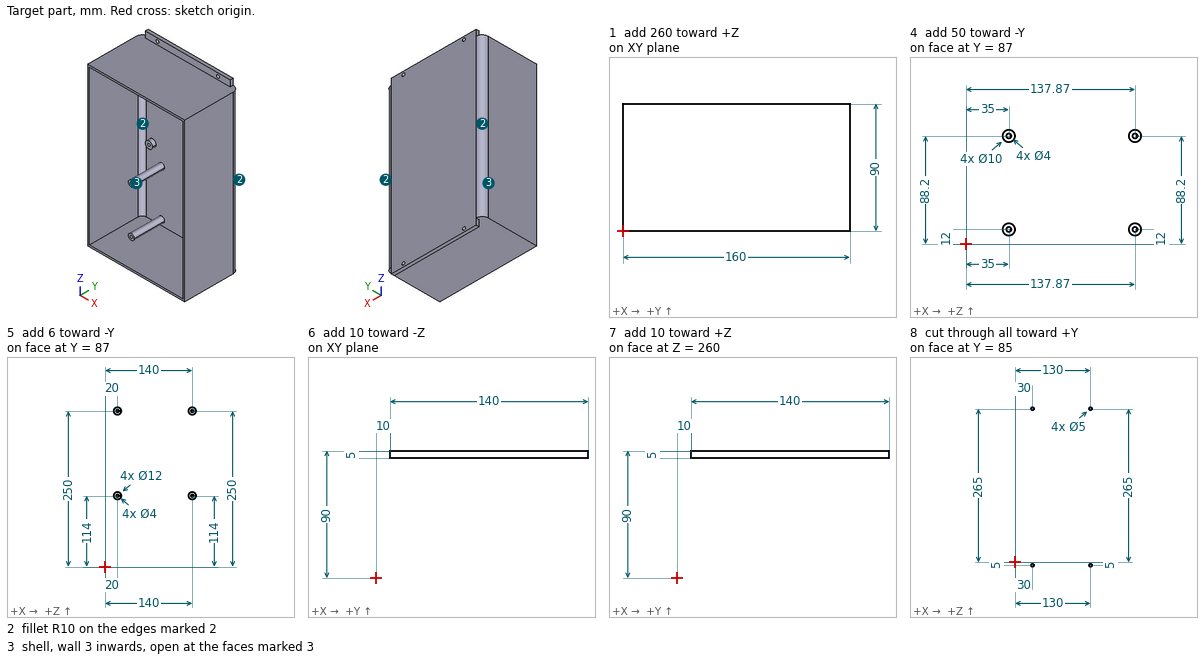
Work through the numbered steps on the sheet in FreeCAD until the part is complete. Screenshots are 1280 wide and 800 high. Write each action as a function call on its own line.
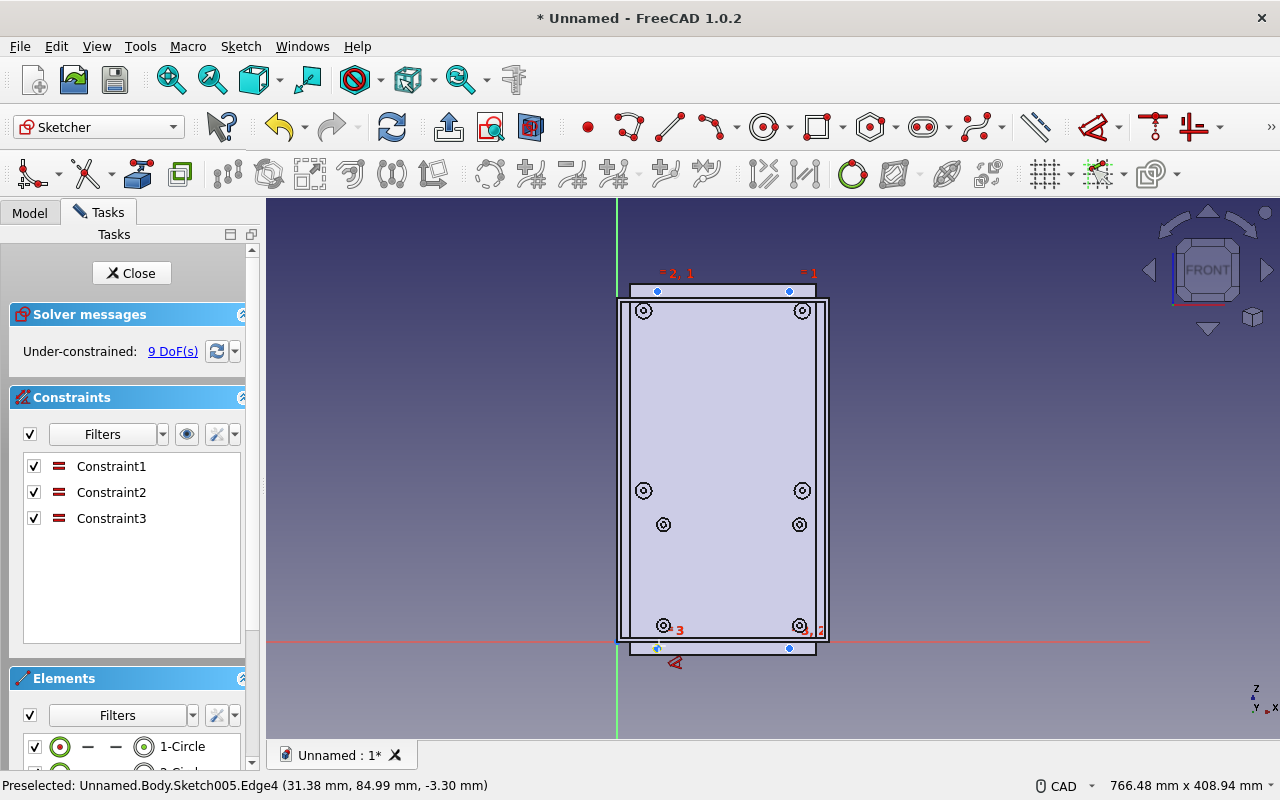
scroll(792, 289, up, 9)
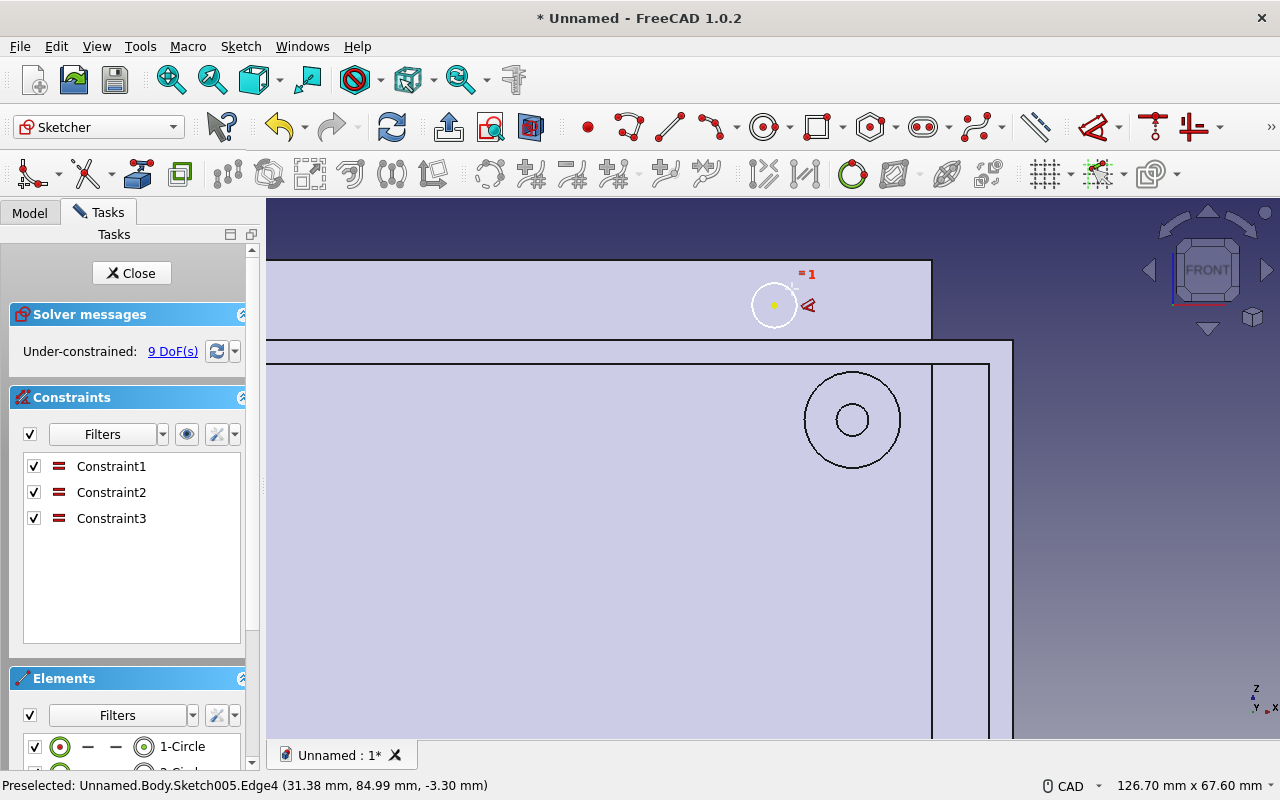
click(790, 290)
click(813, 267)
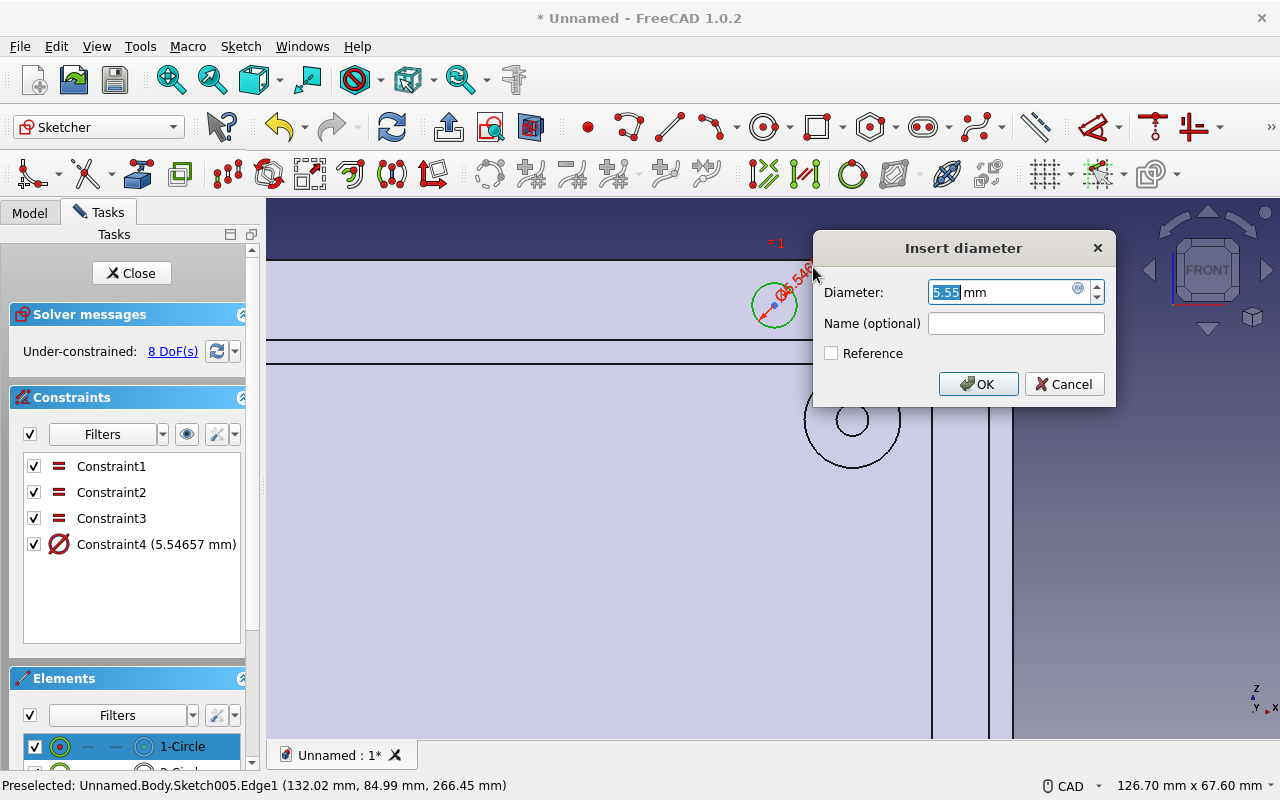
text(5)
key(Return)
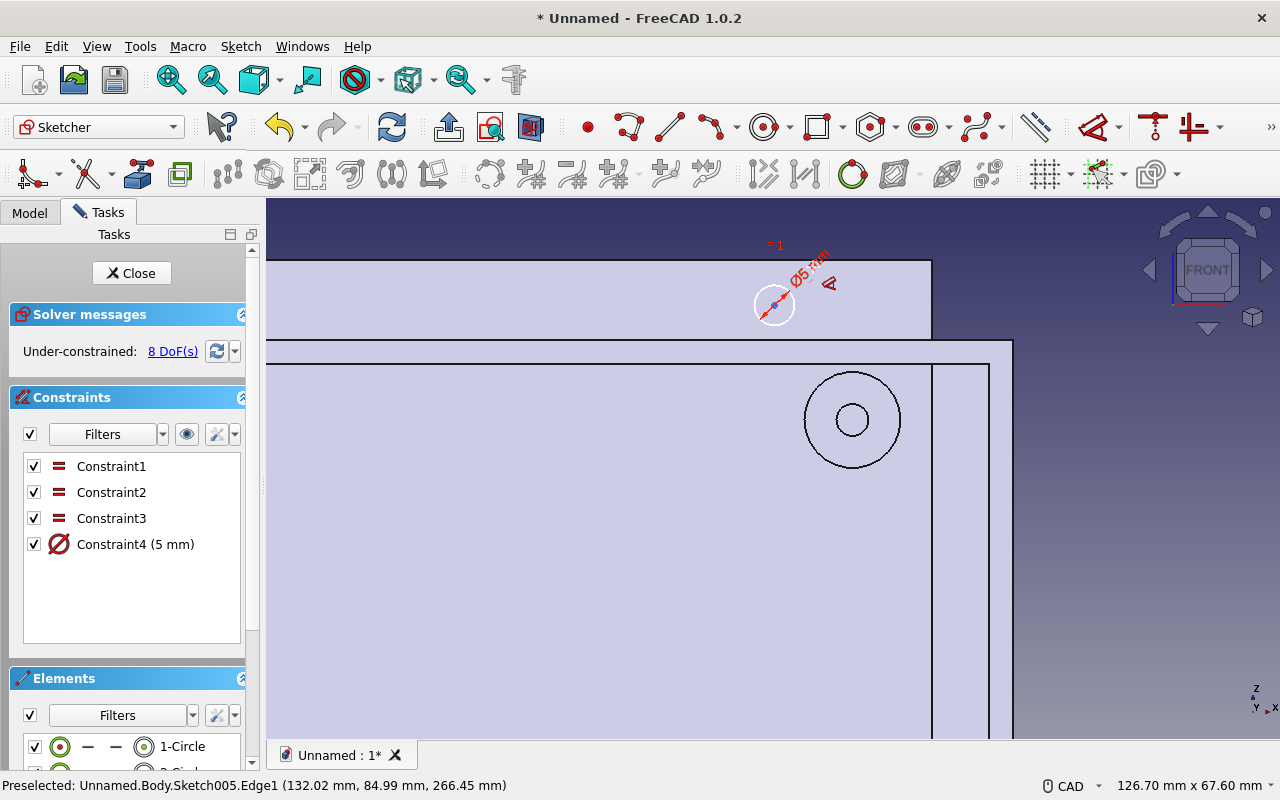
scroll(792, 288, down, 9)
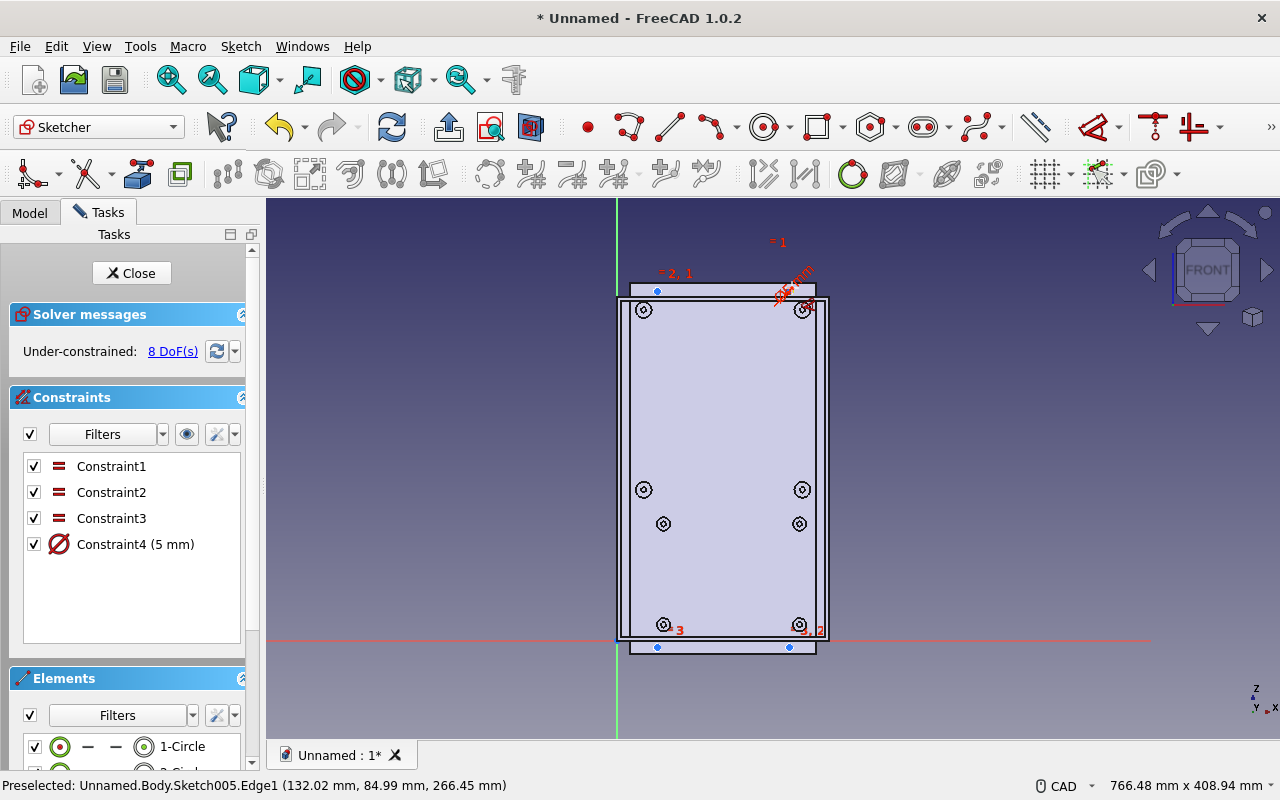
scroll(789, 648, up, 9)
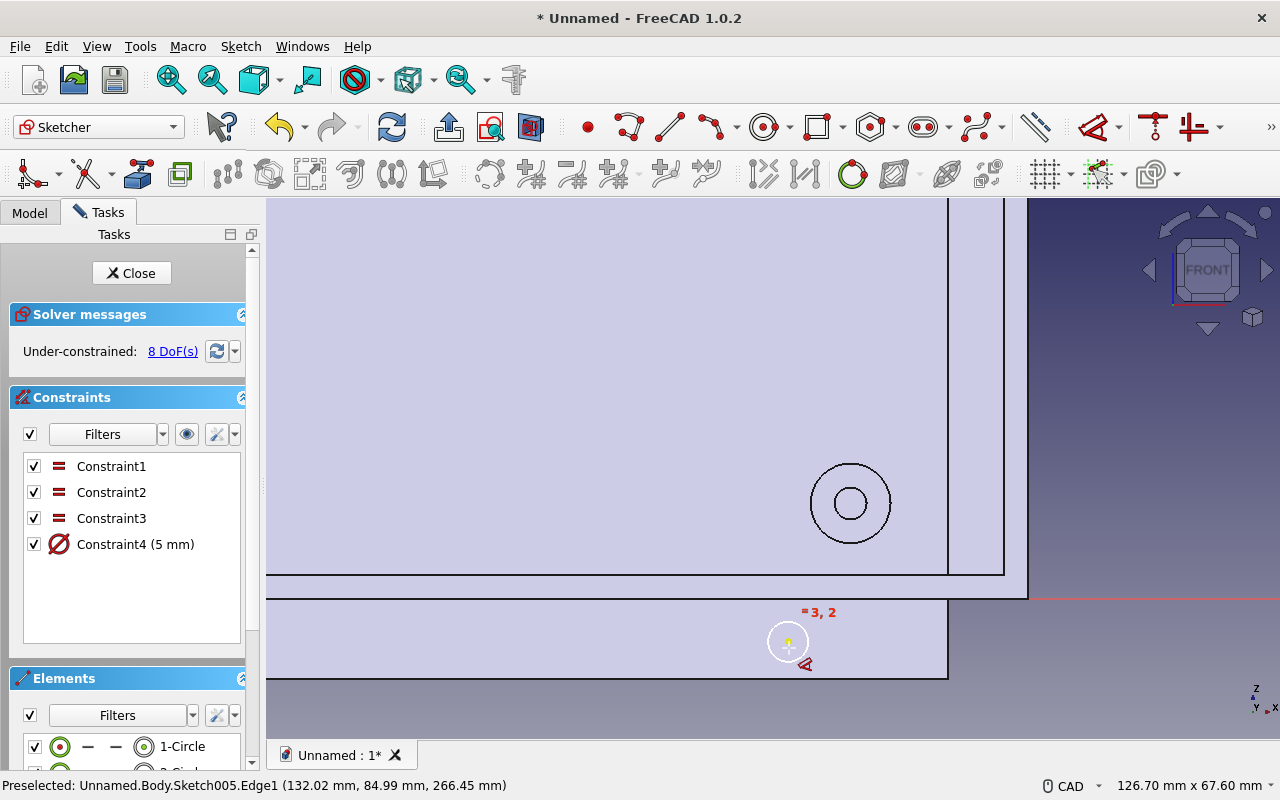
click(788, 642)
click(822, 621)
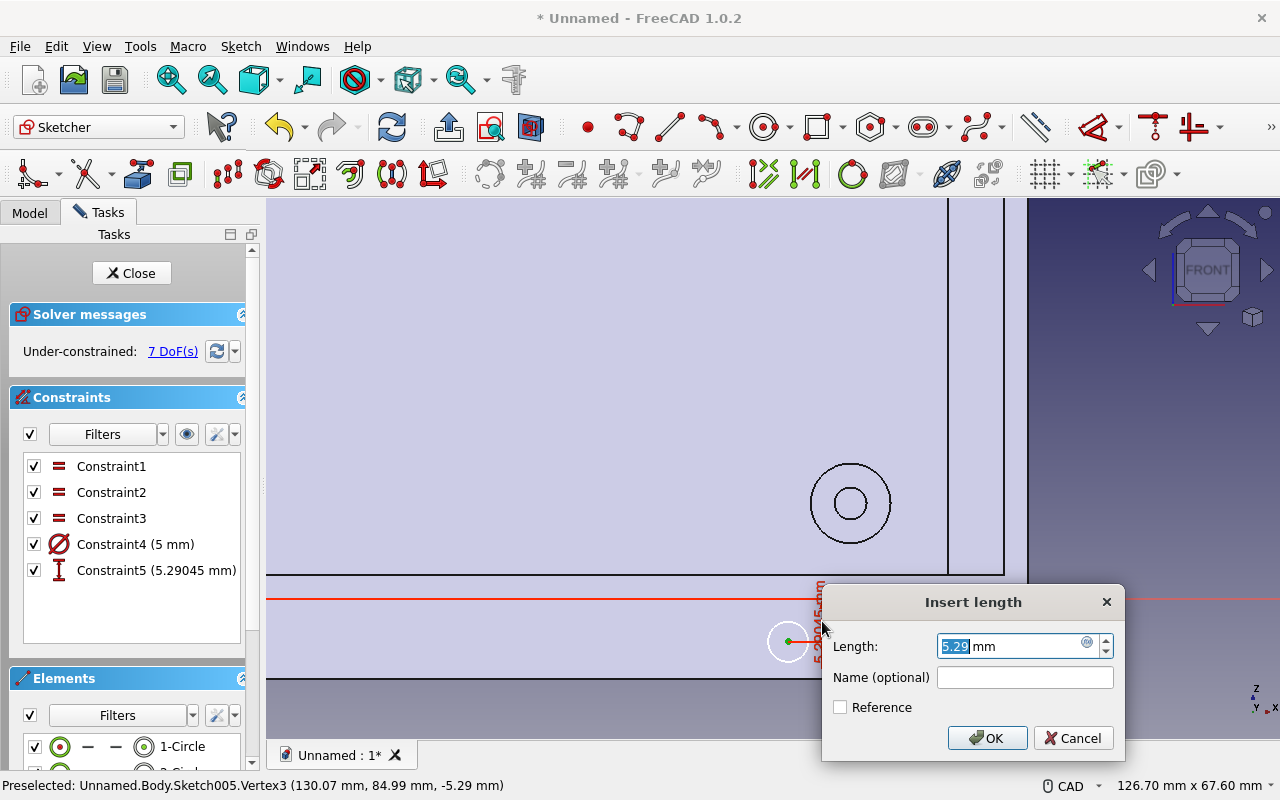
text(5)
key(Return)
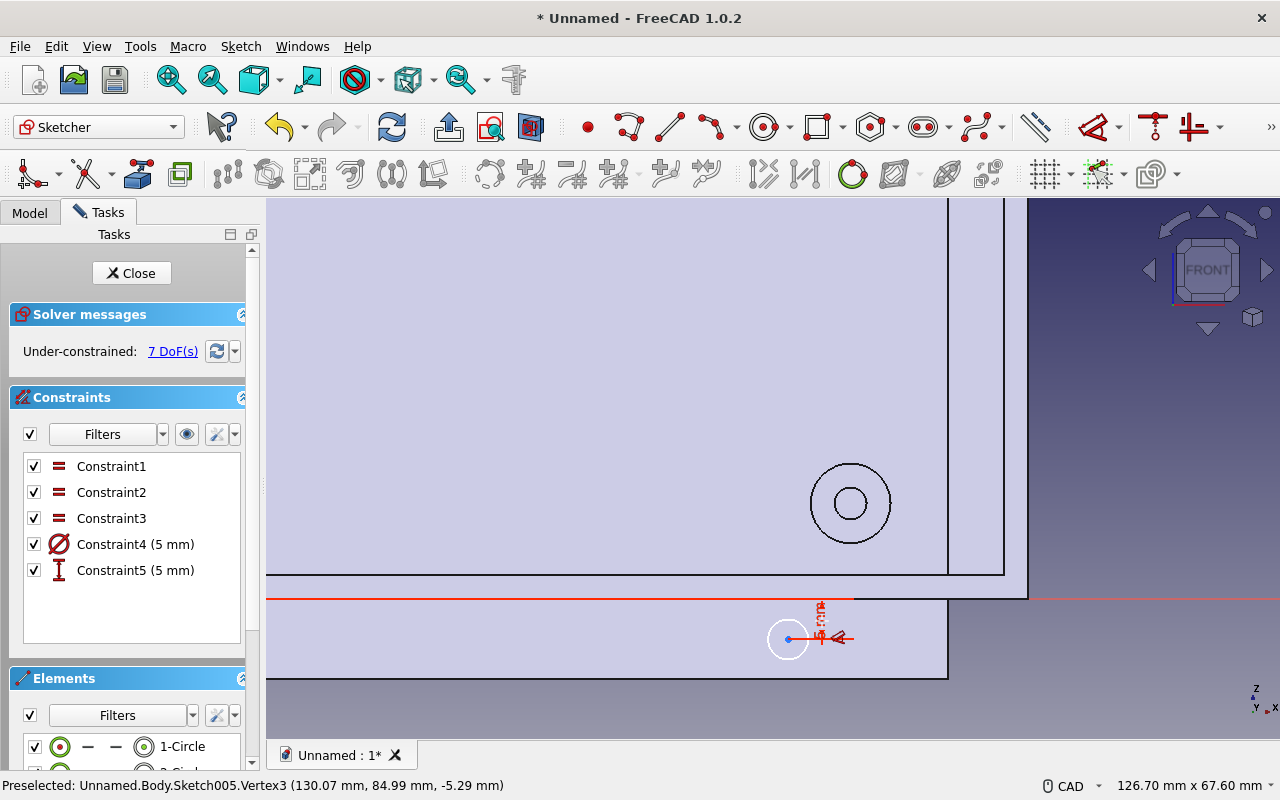
scroll(789, 649, down, 9)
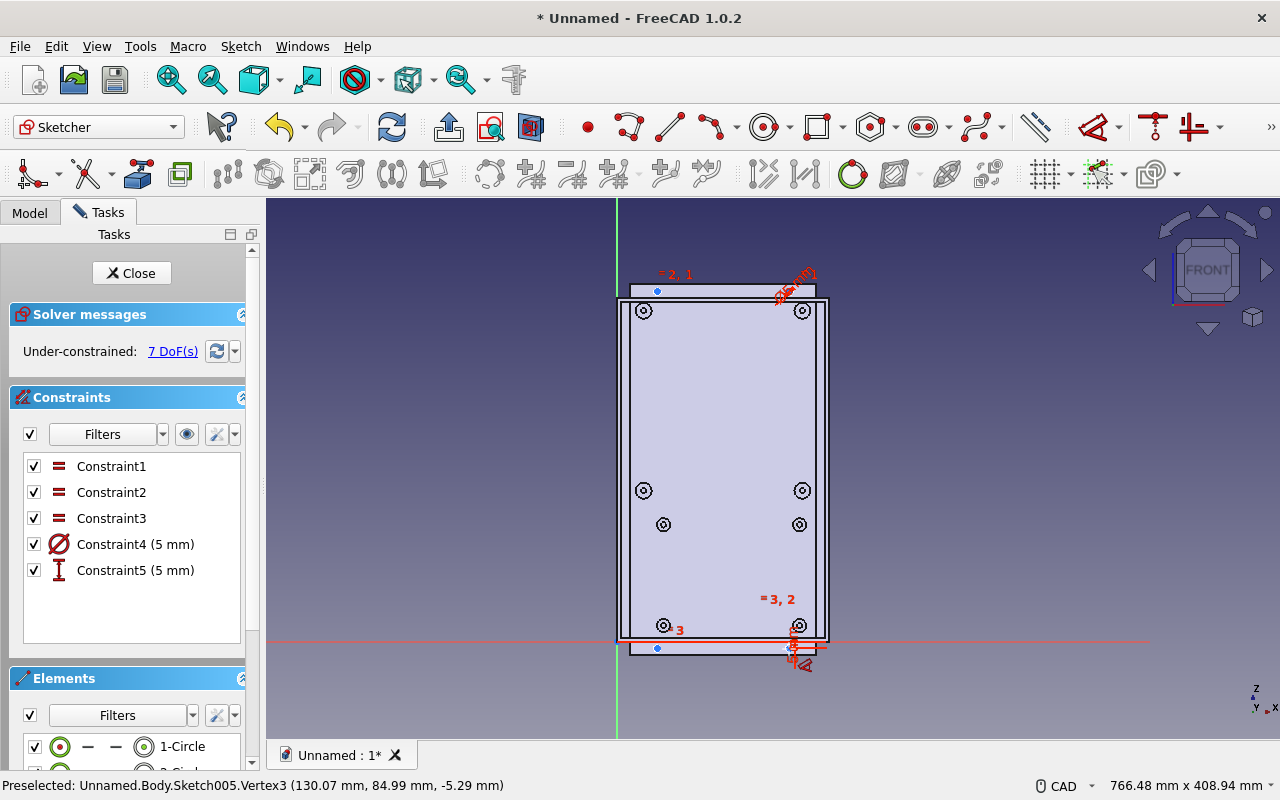
scroll(657, 649, up, 9)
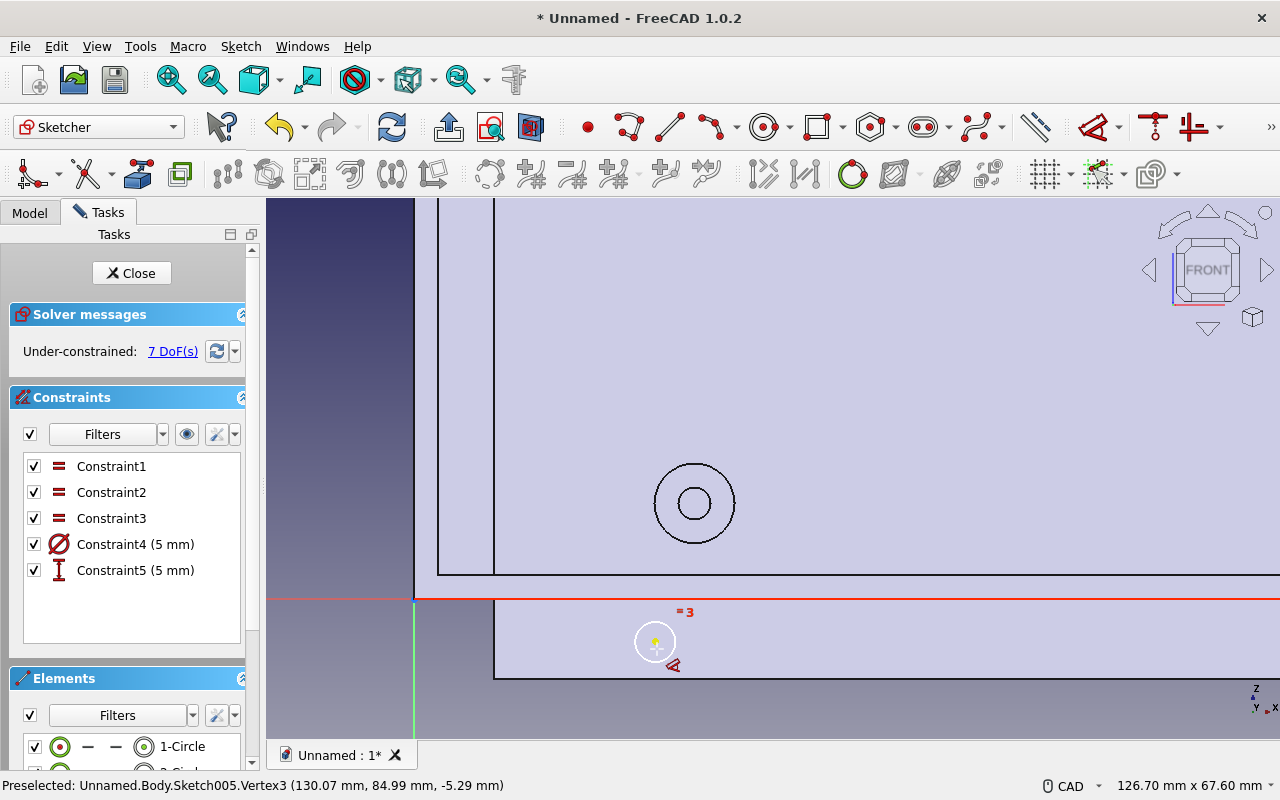
click(655, 642)
click(380, 621)